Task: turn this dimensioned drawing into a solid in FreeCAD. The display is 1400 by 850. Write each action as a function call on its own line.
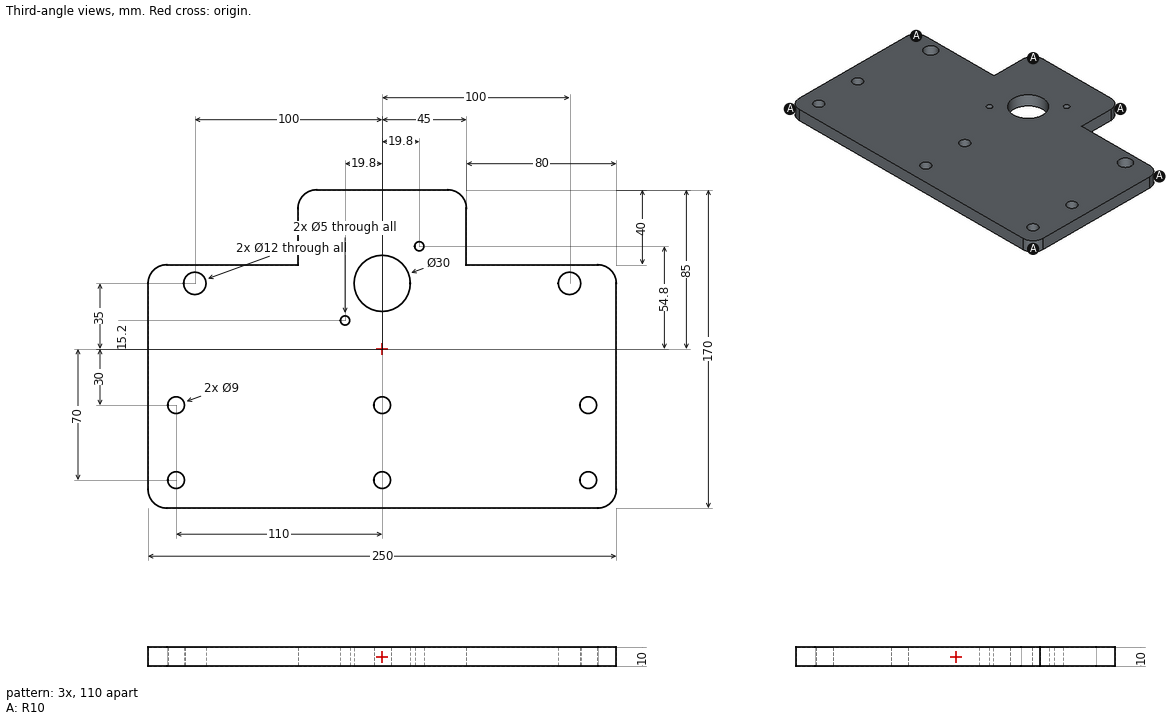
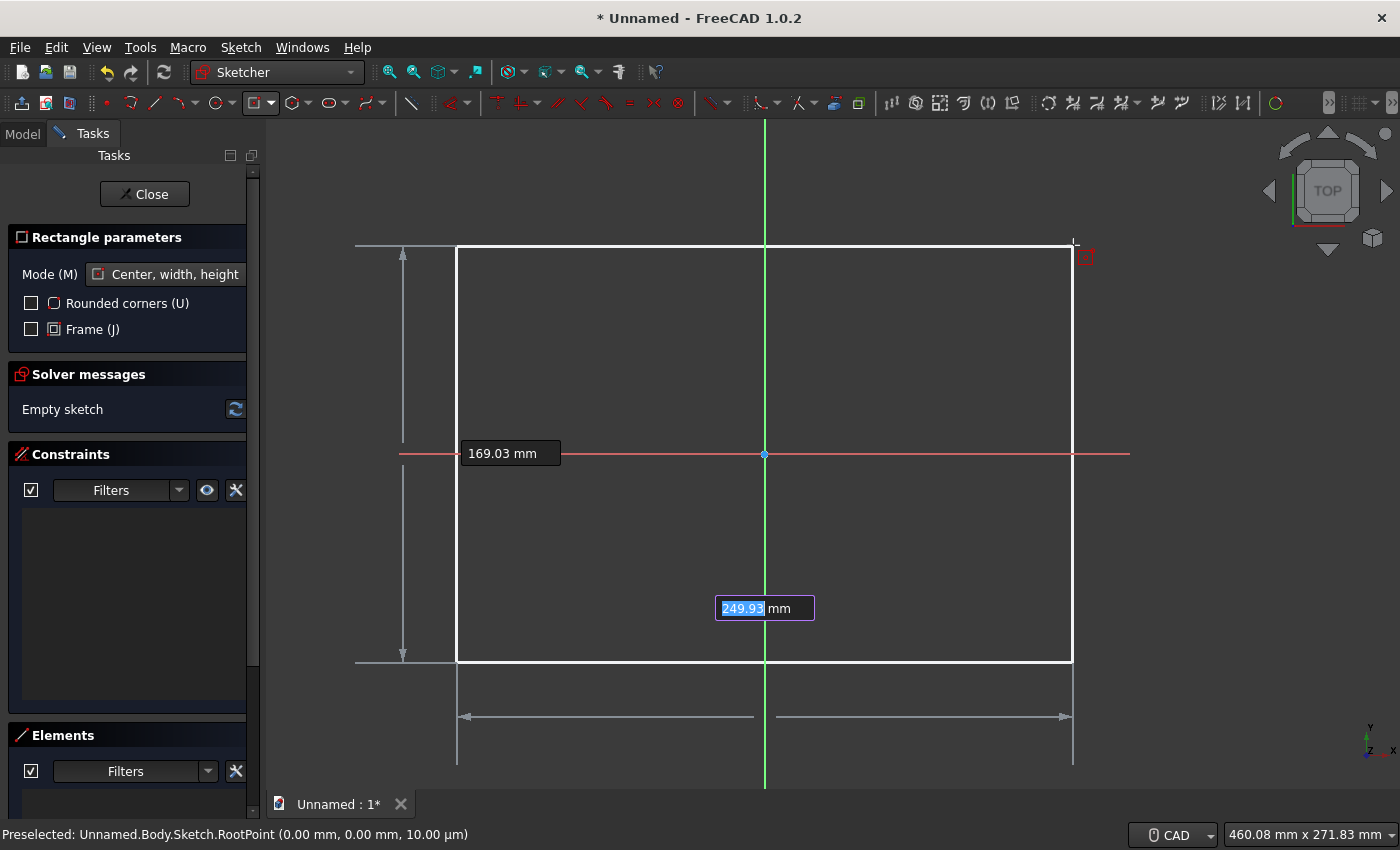
text(250)
key(Tab)
text(170)
key(Return)
key(Escape)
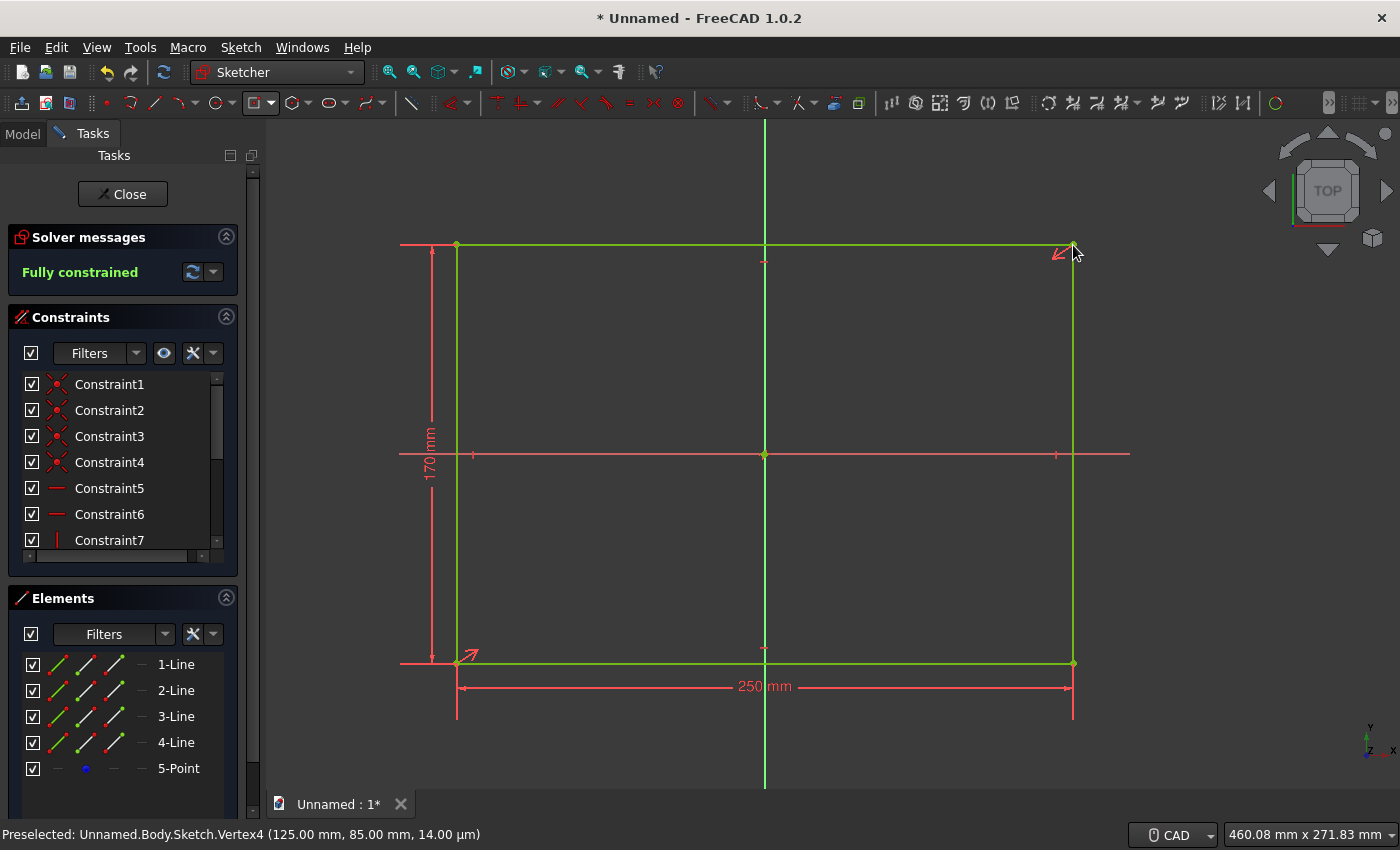
click(123, 194)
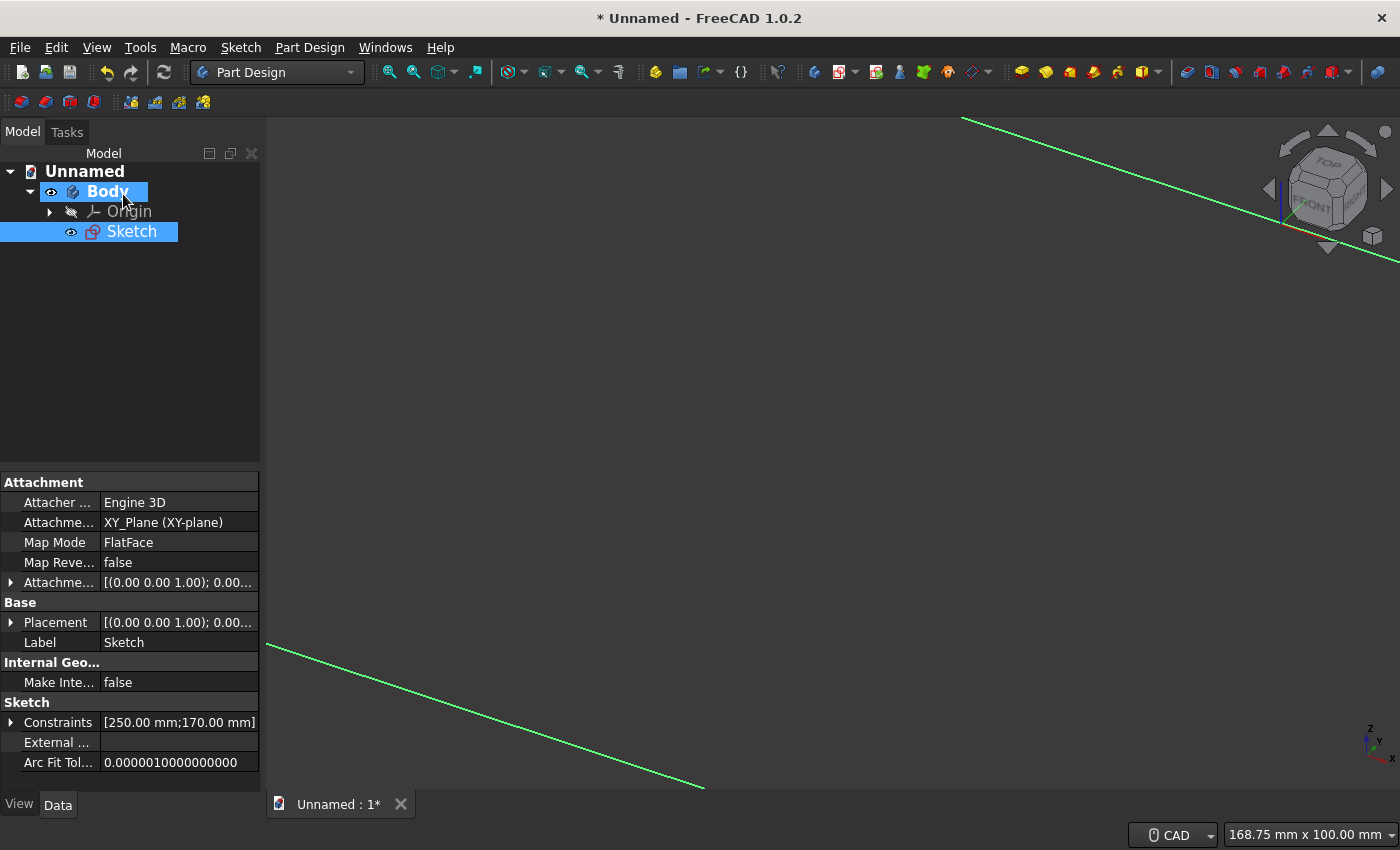
click(1022, 72)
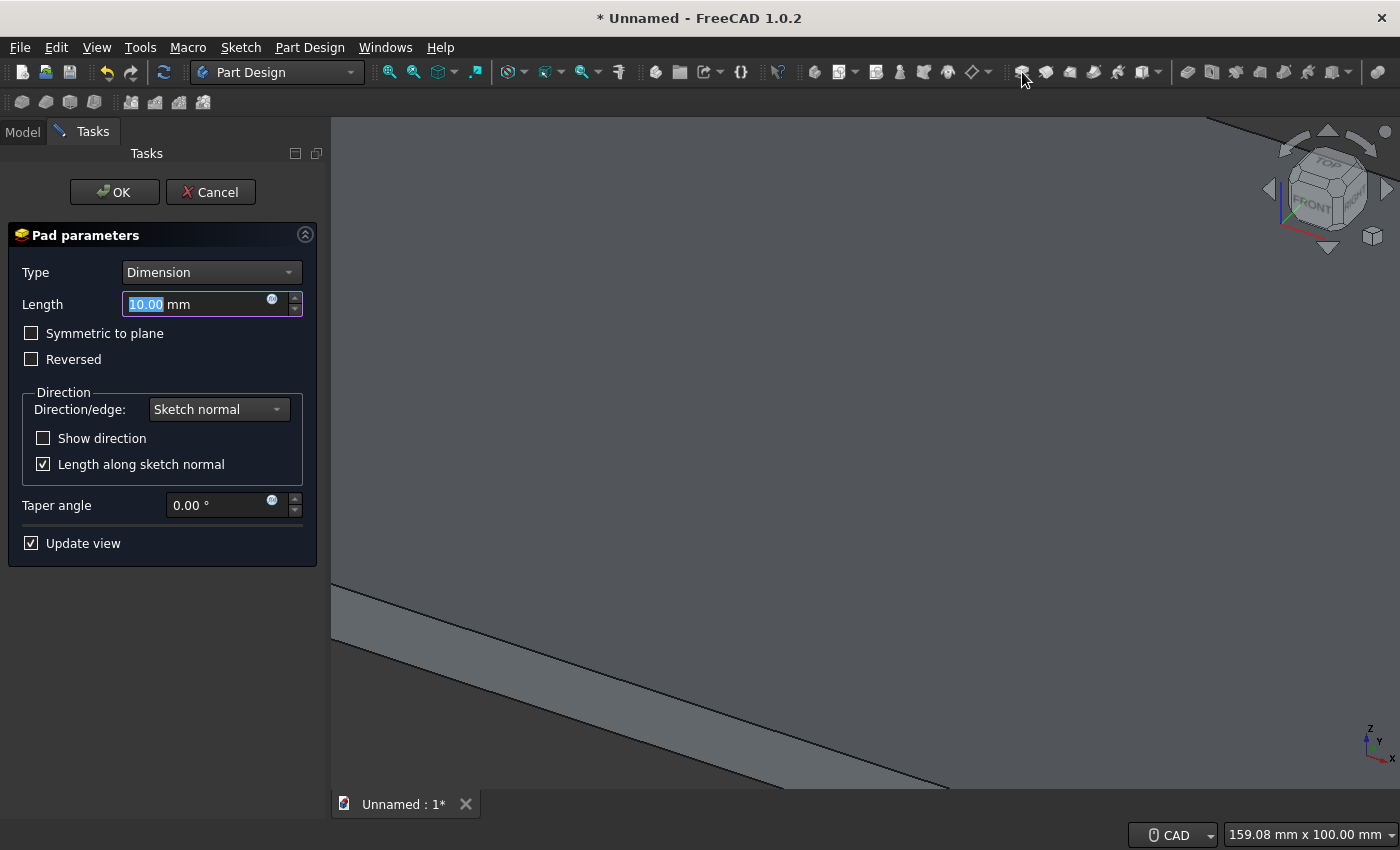
text(10)
key(Tab)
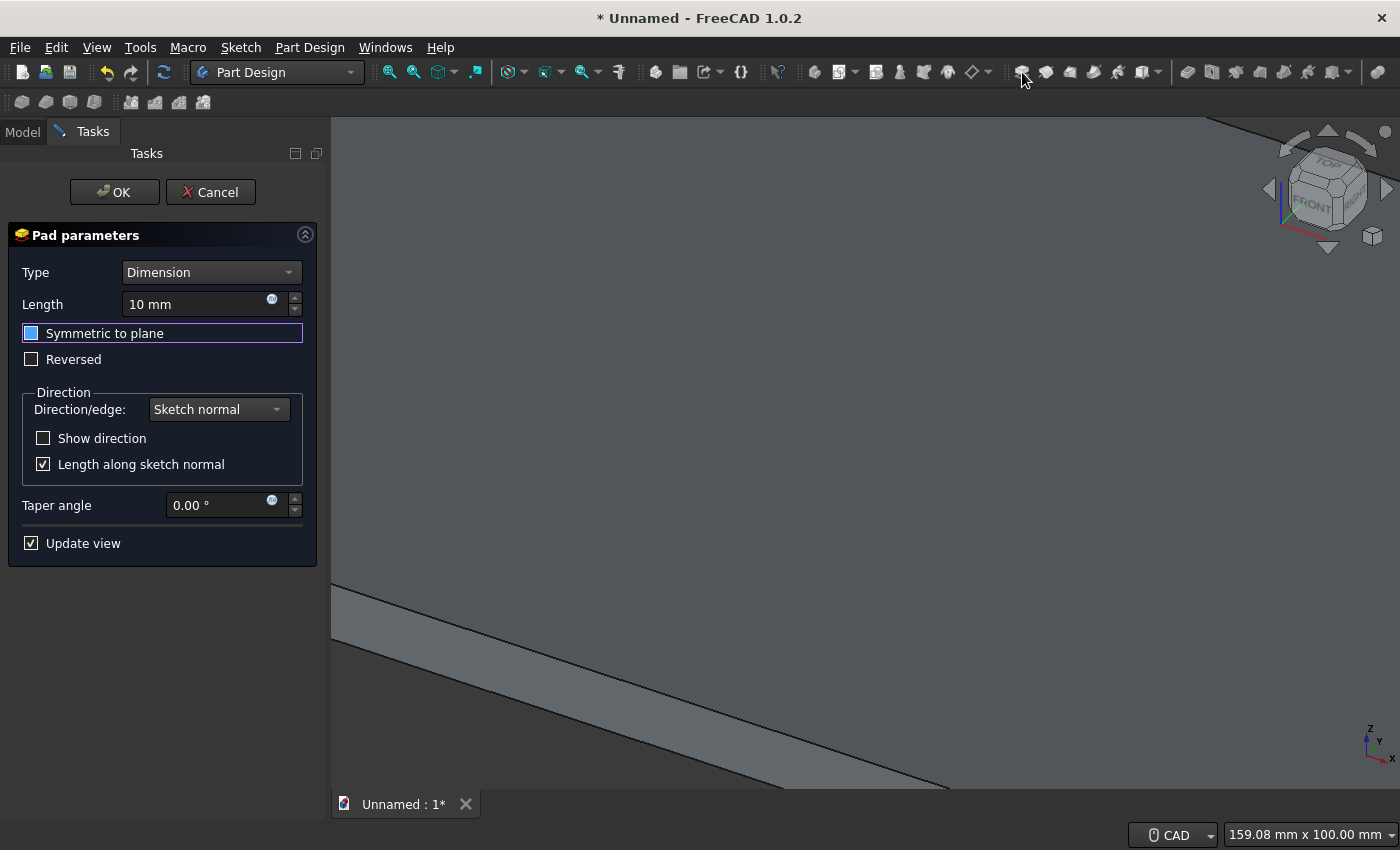
click(30, 333)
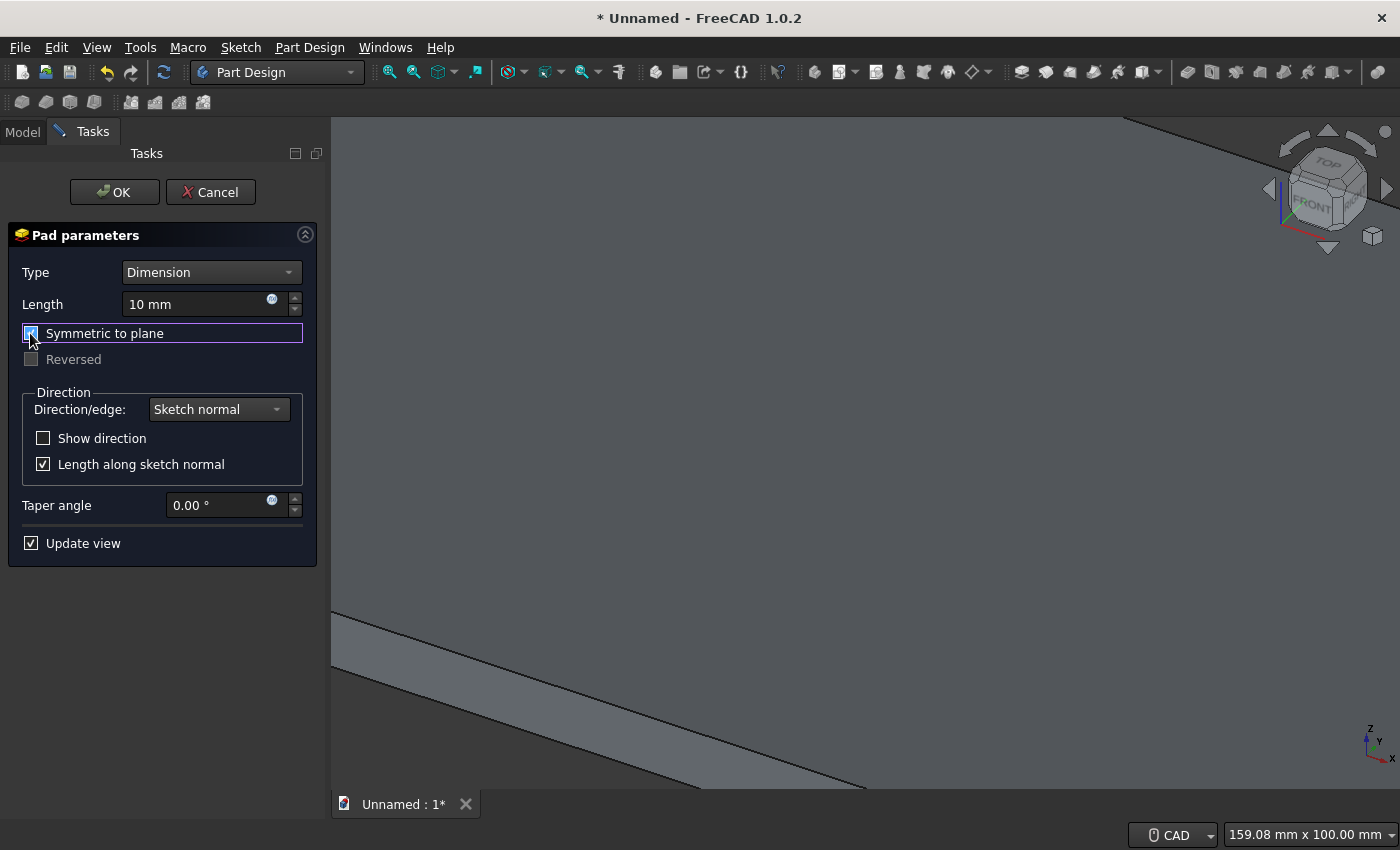
click(115, 192)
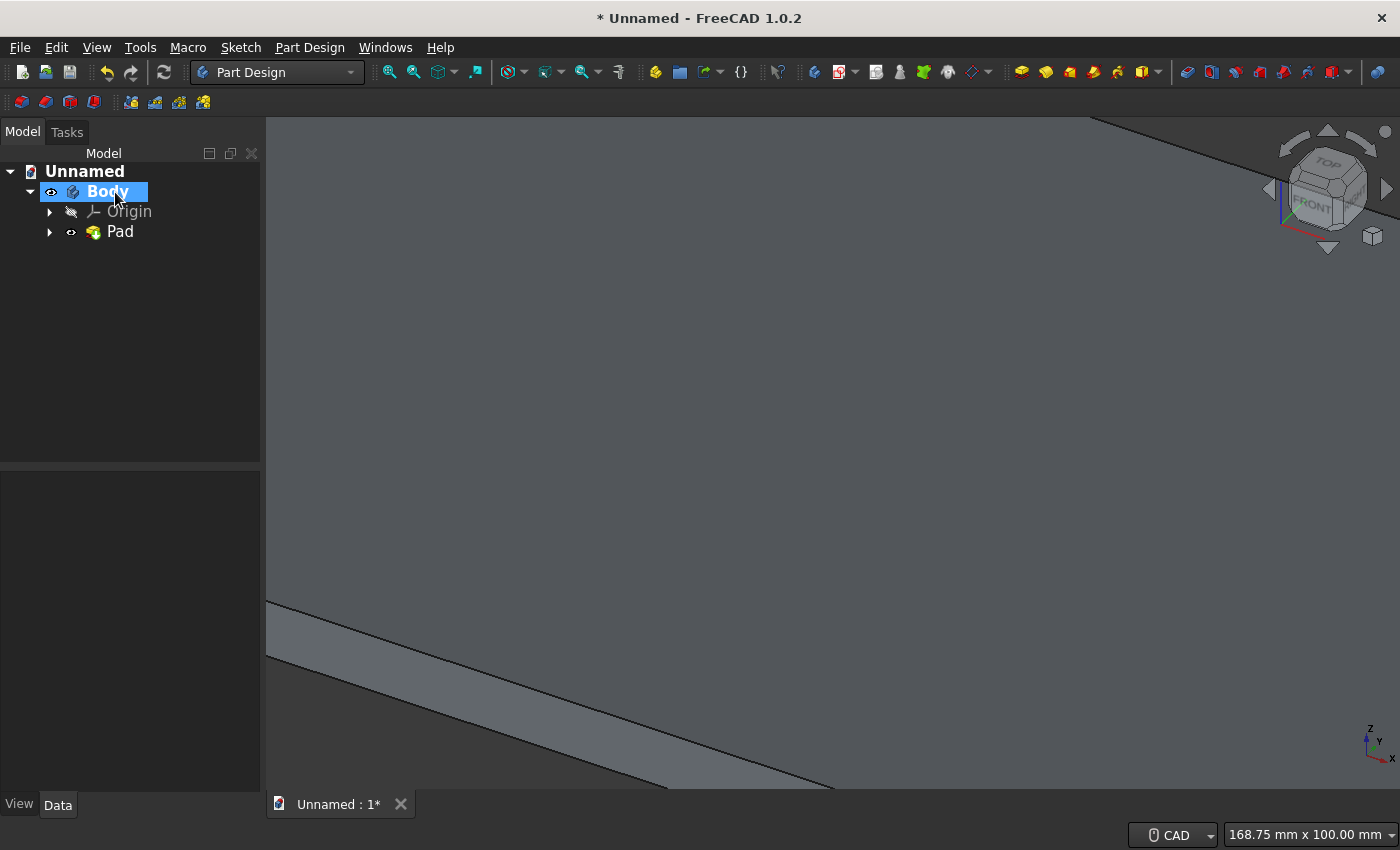
click(390, 72)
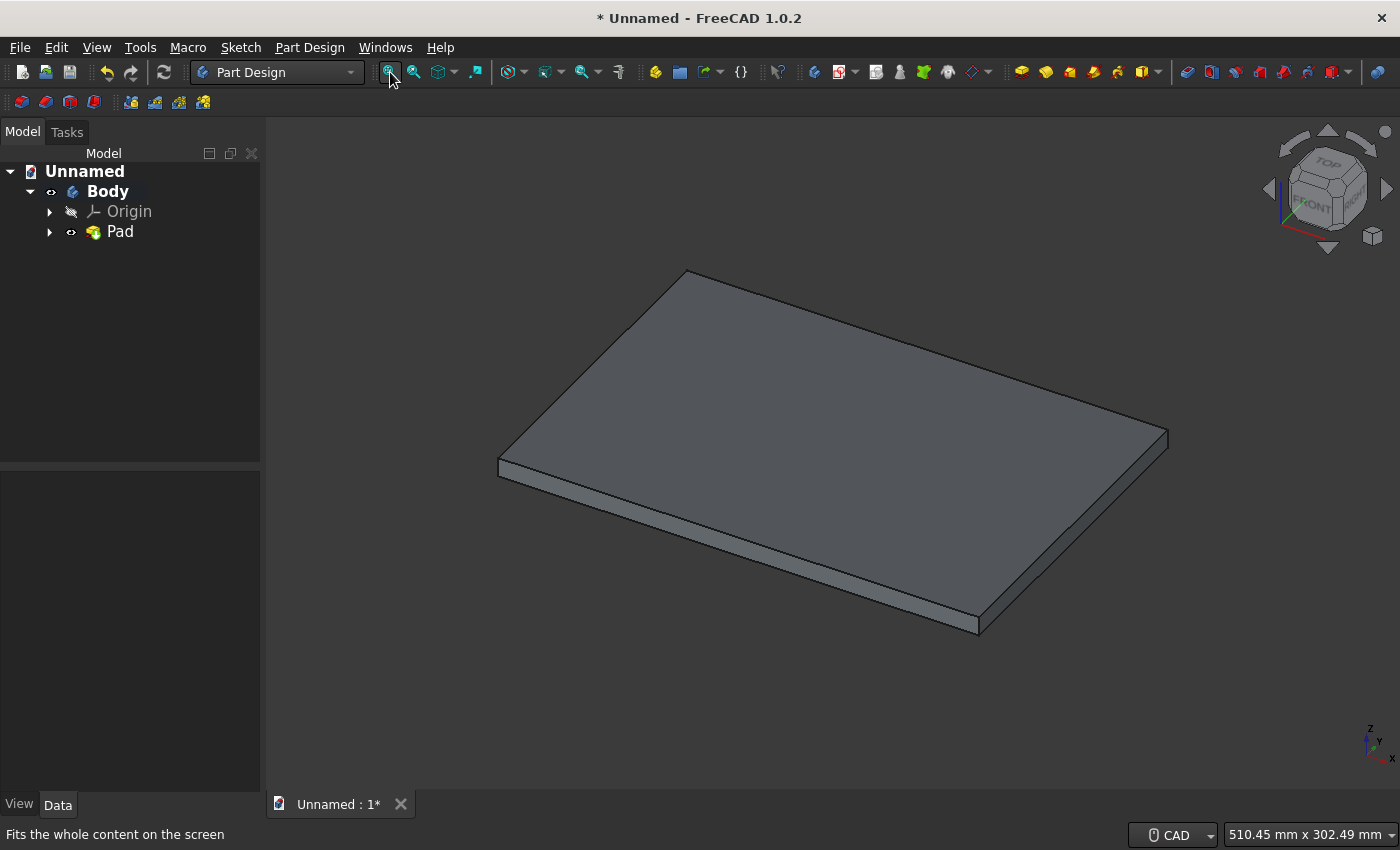
click(902, 466)